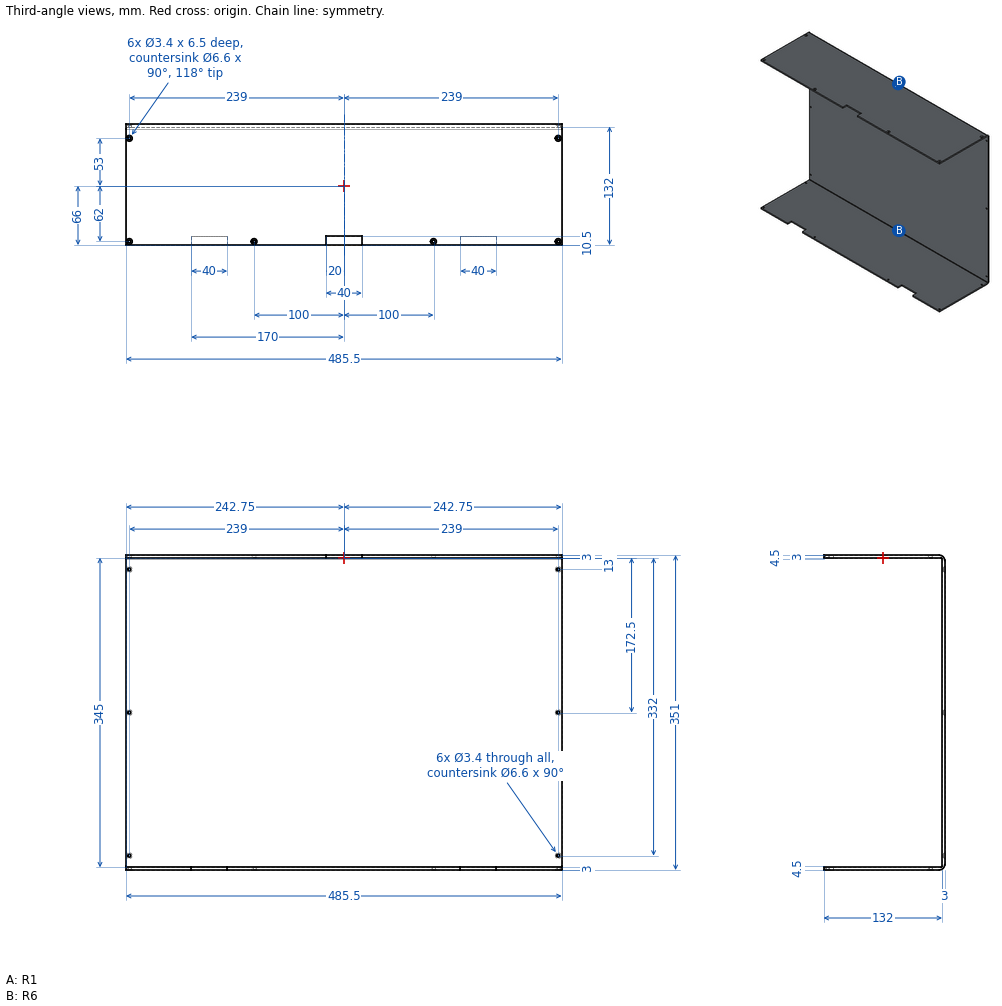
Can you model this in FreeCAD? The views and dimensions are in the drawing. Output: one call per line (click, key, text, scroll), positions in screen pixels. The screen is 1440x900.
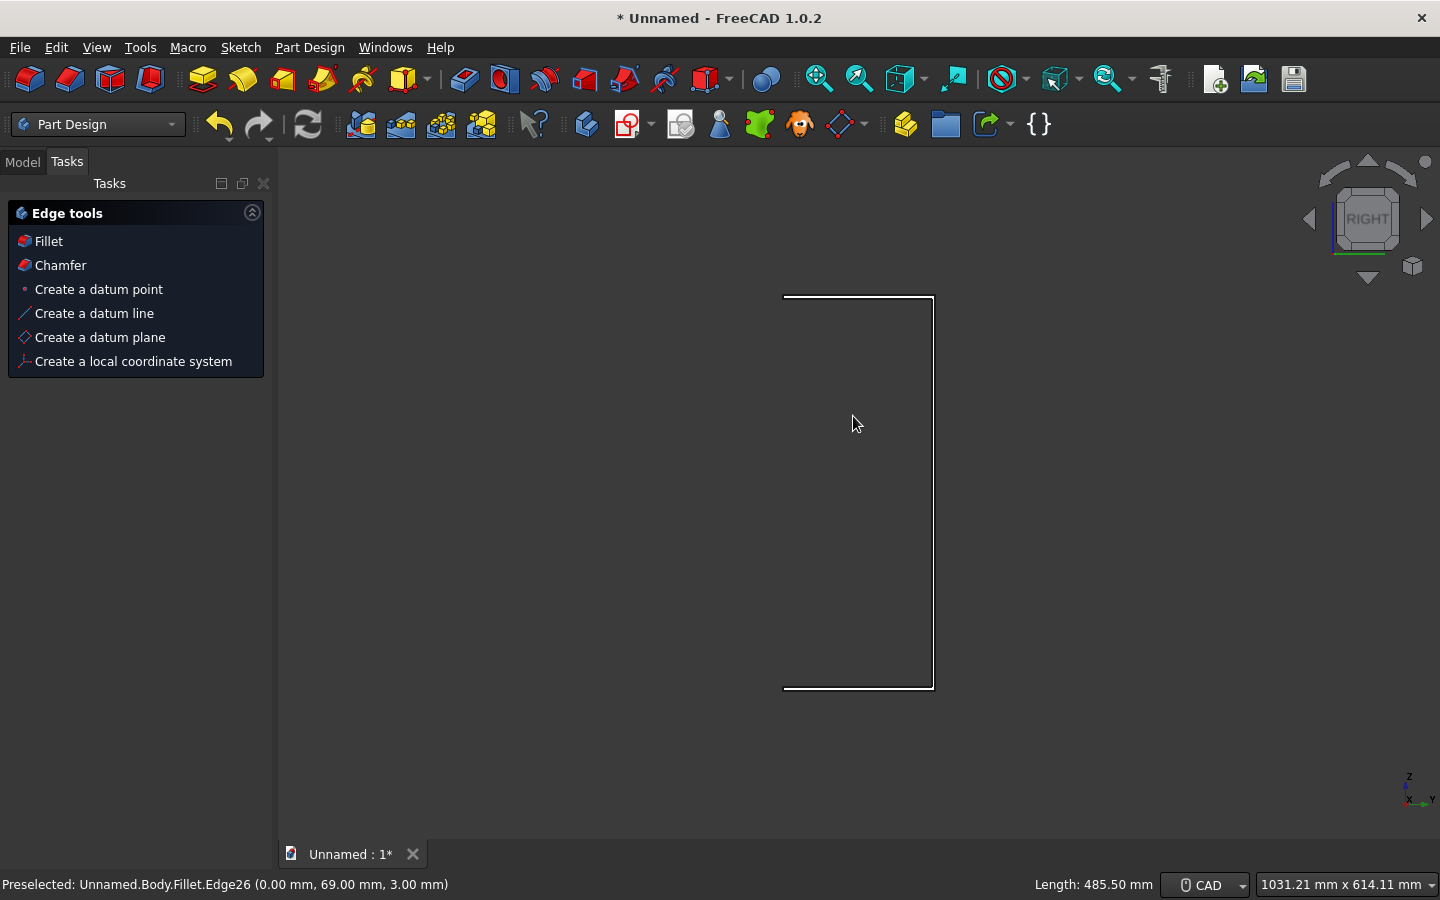
key(5)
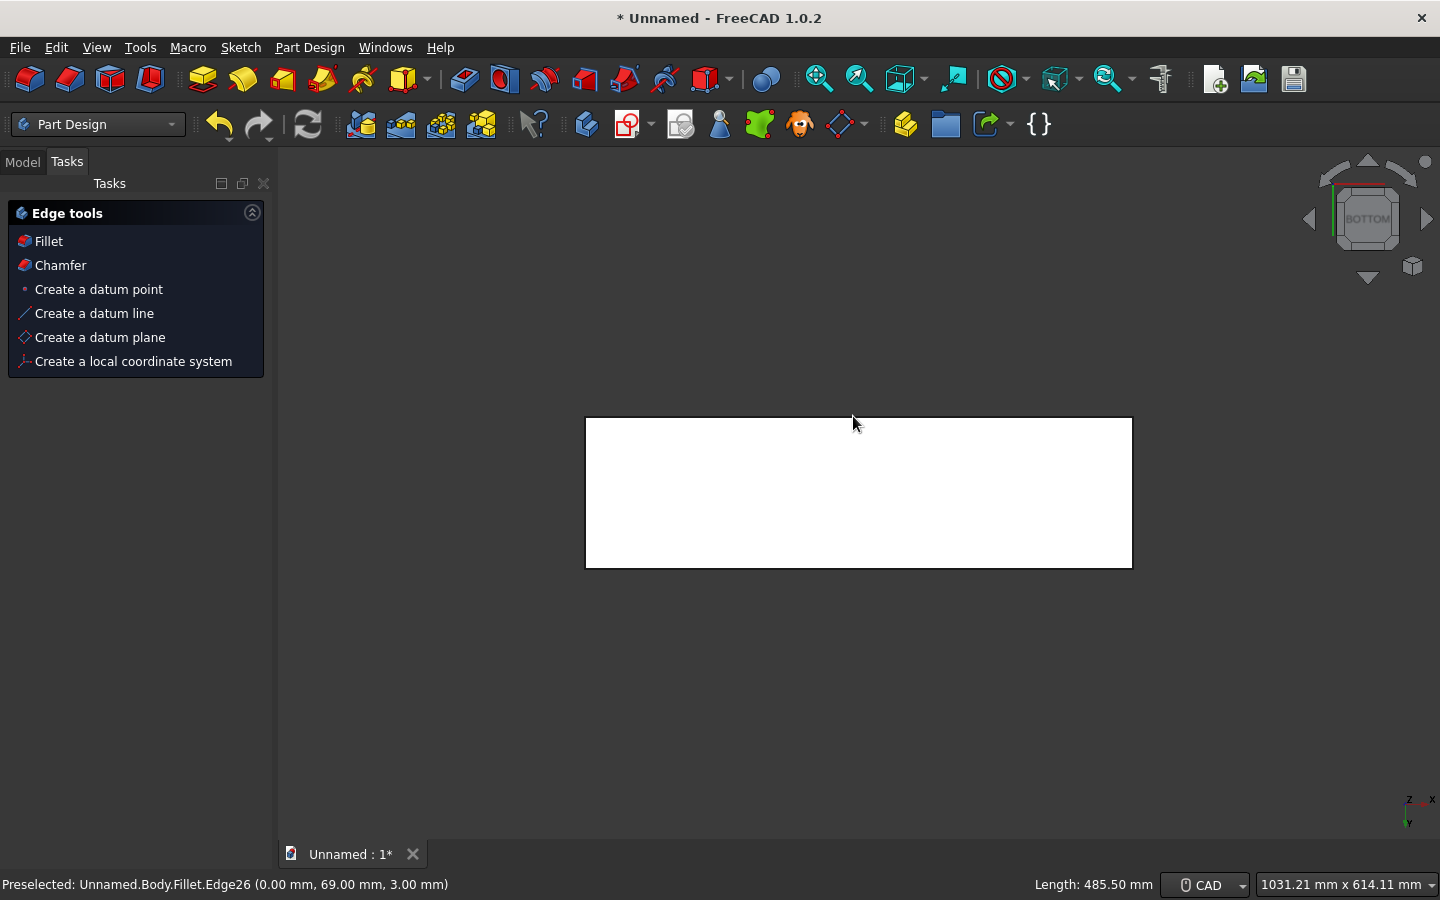
click(859, 568, ctrl)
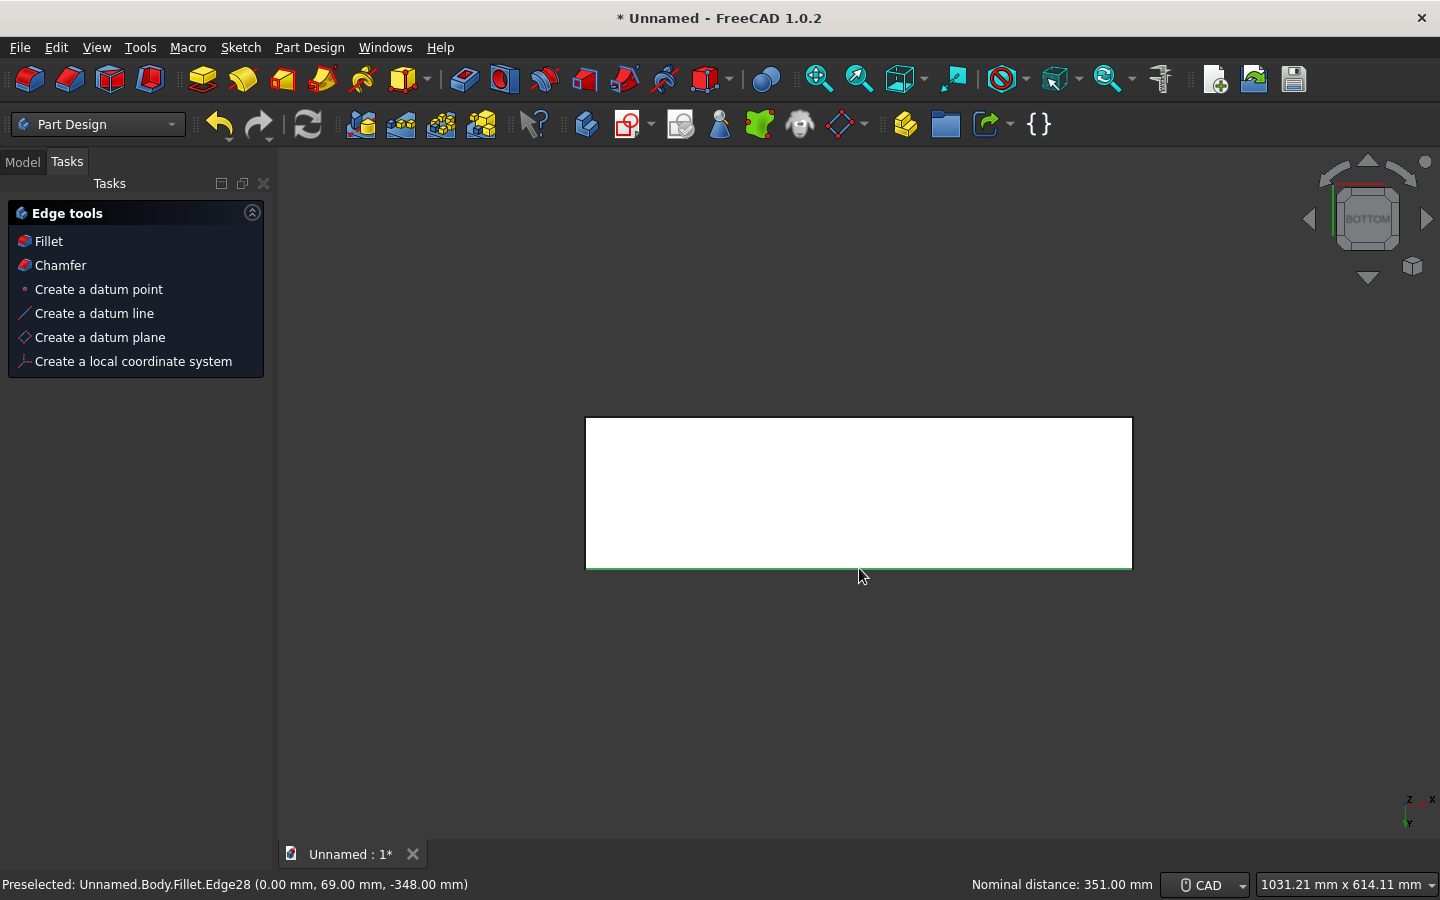
click(30, 80)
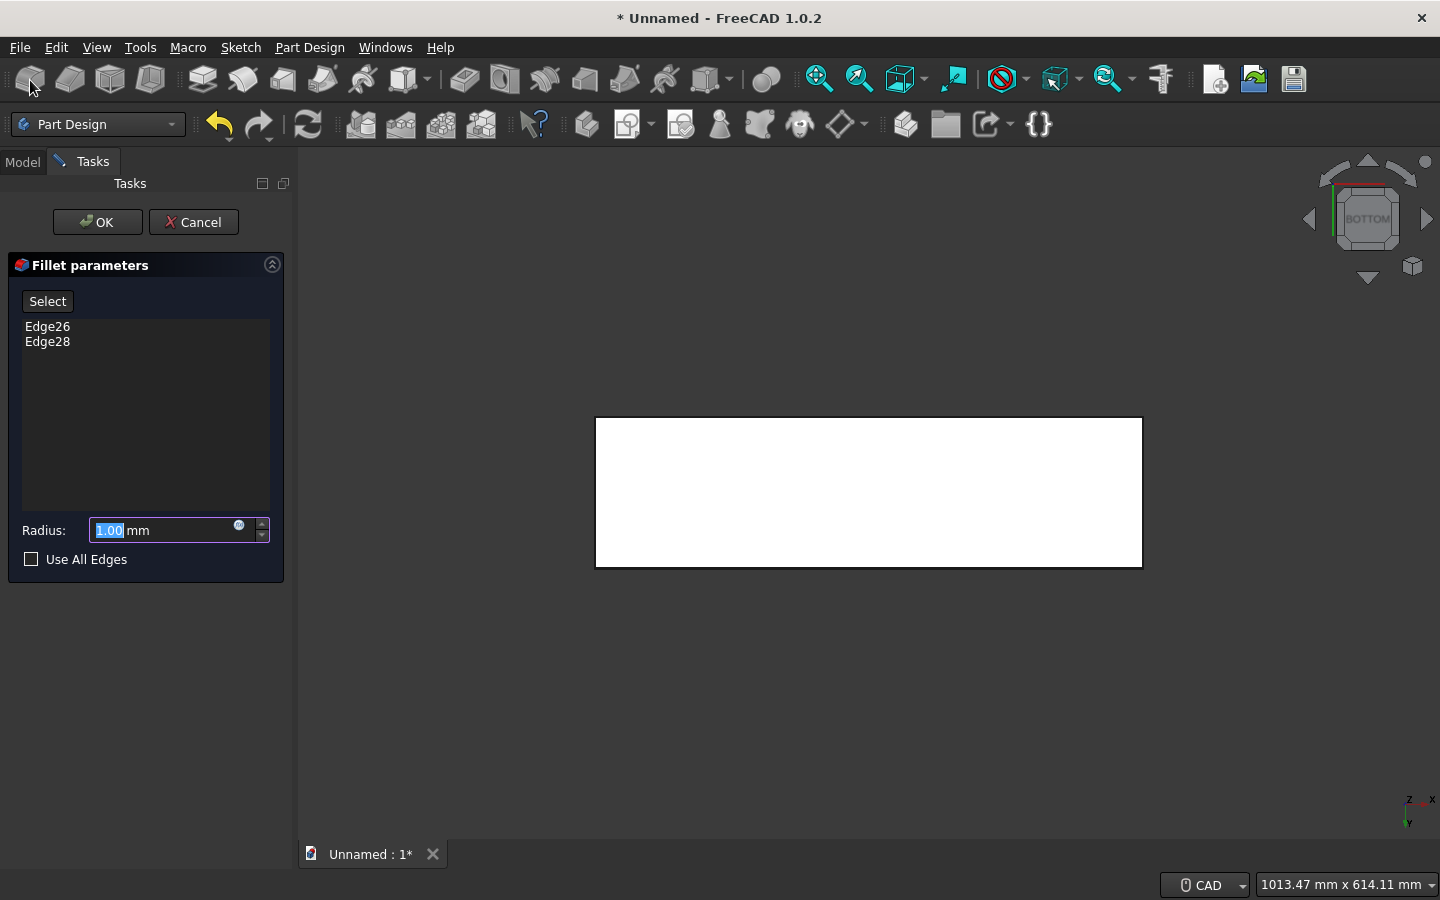
text(6)
key(Tab)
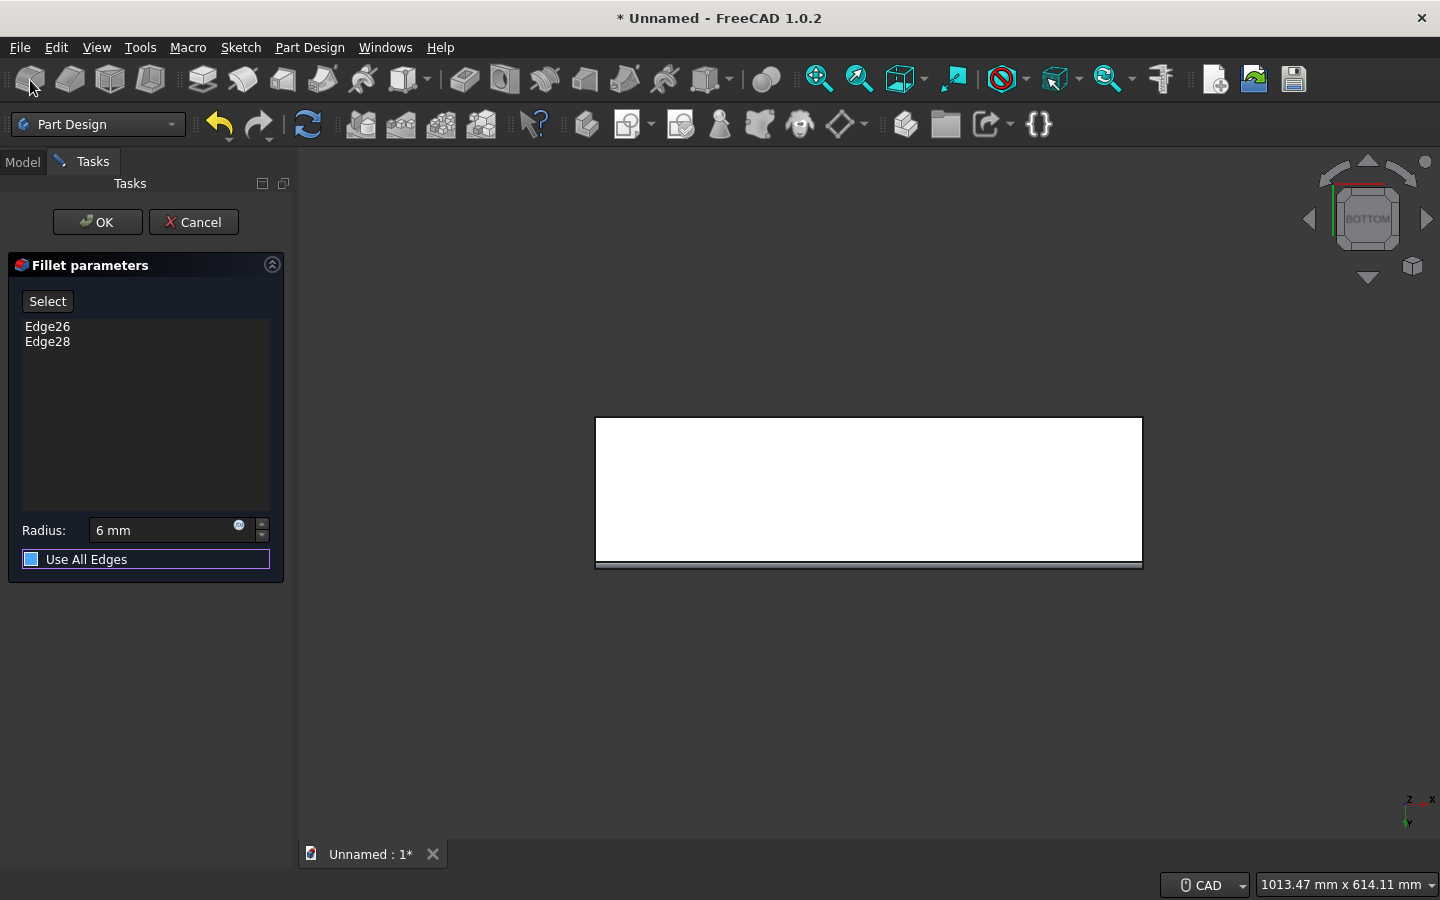
click(98, 222)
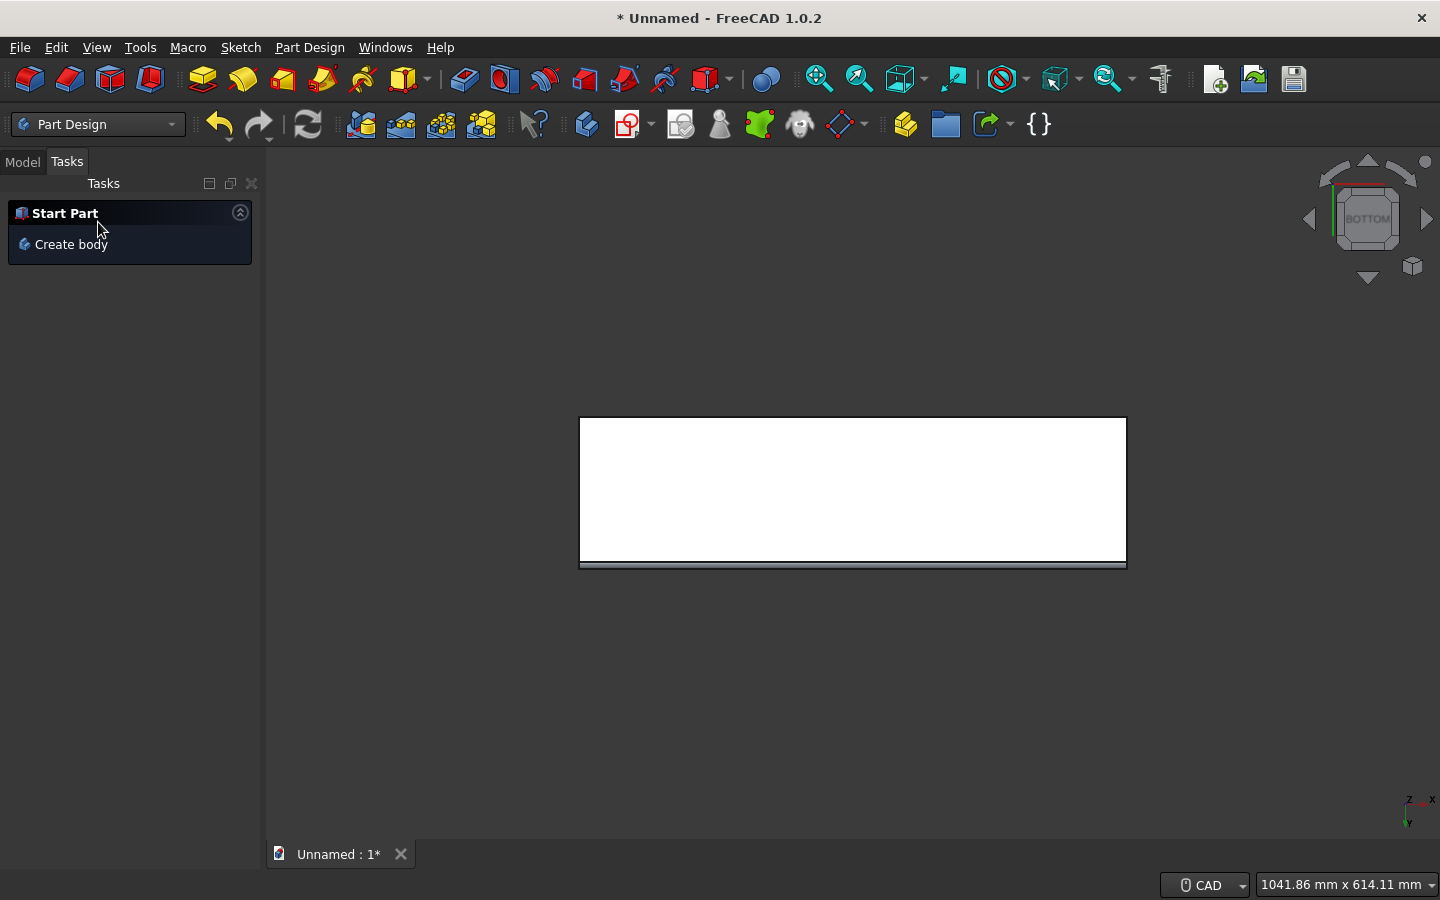
key(0)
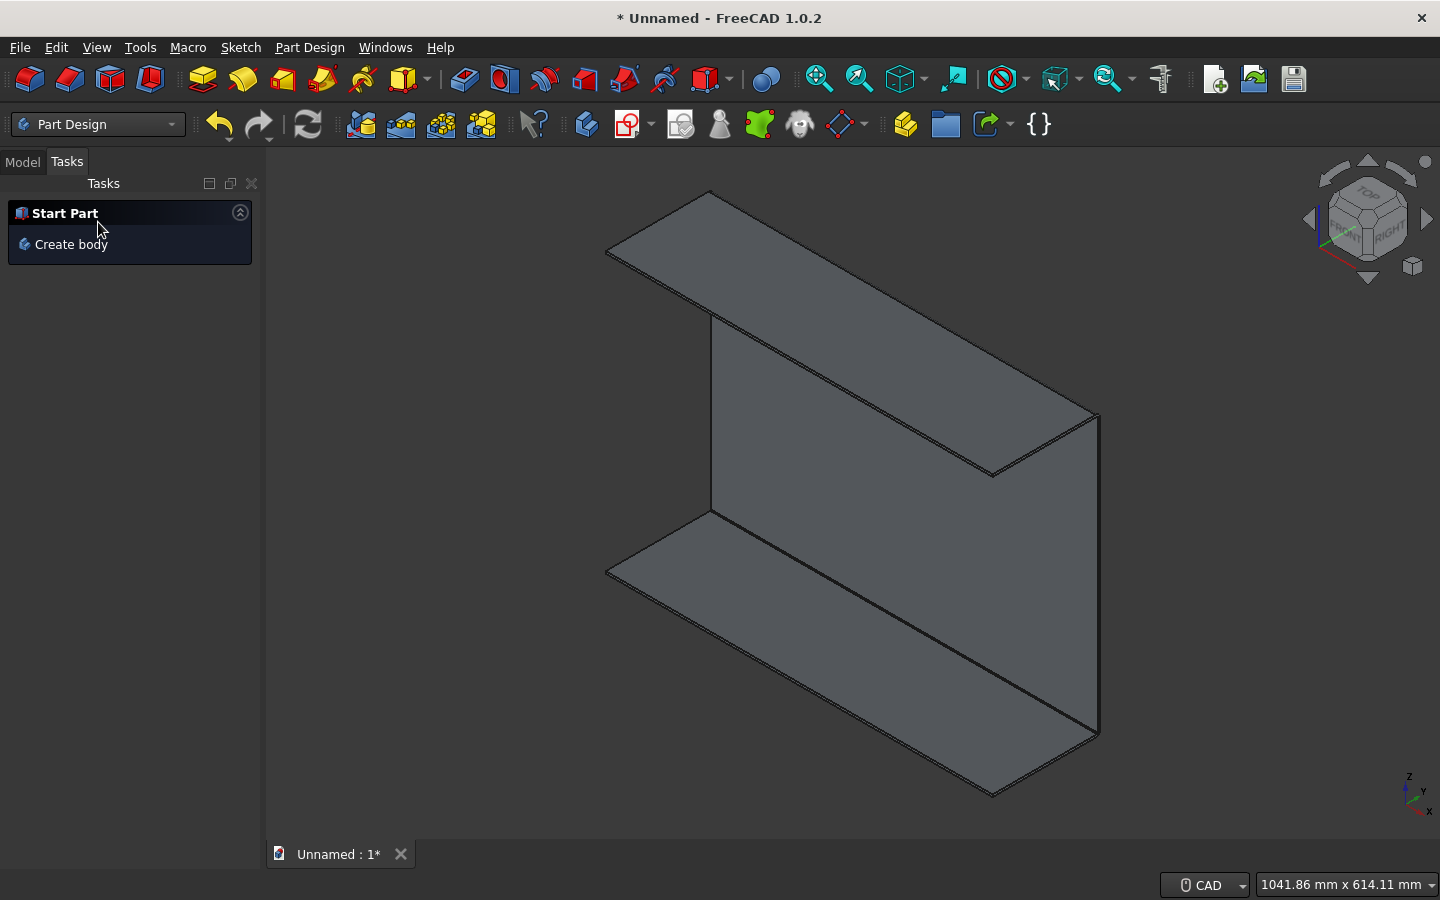
click(961, 396)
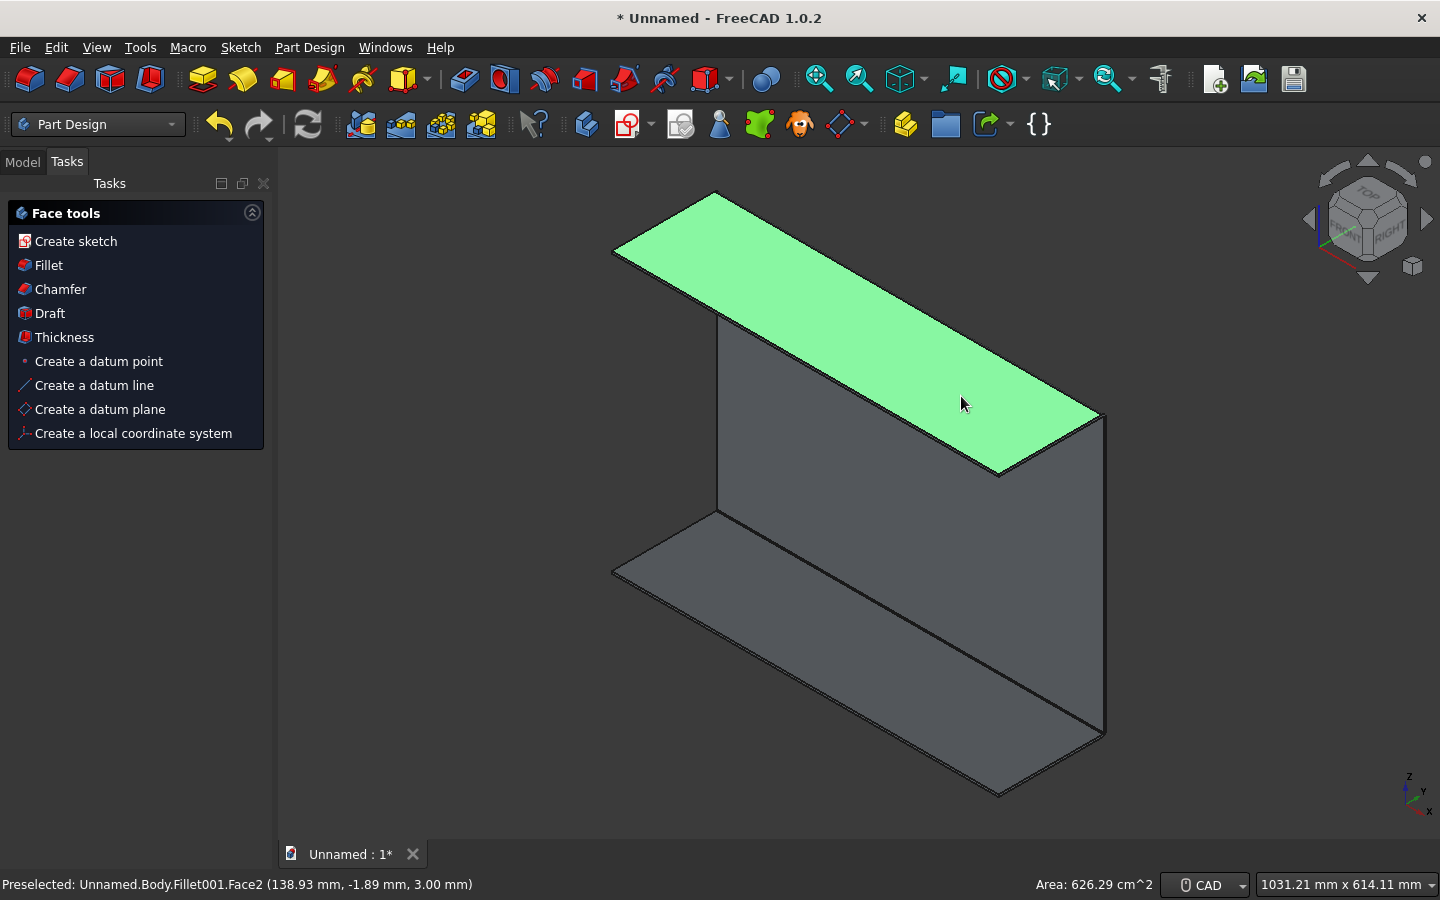
click(628, 124)